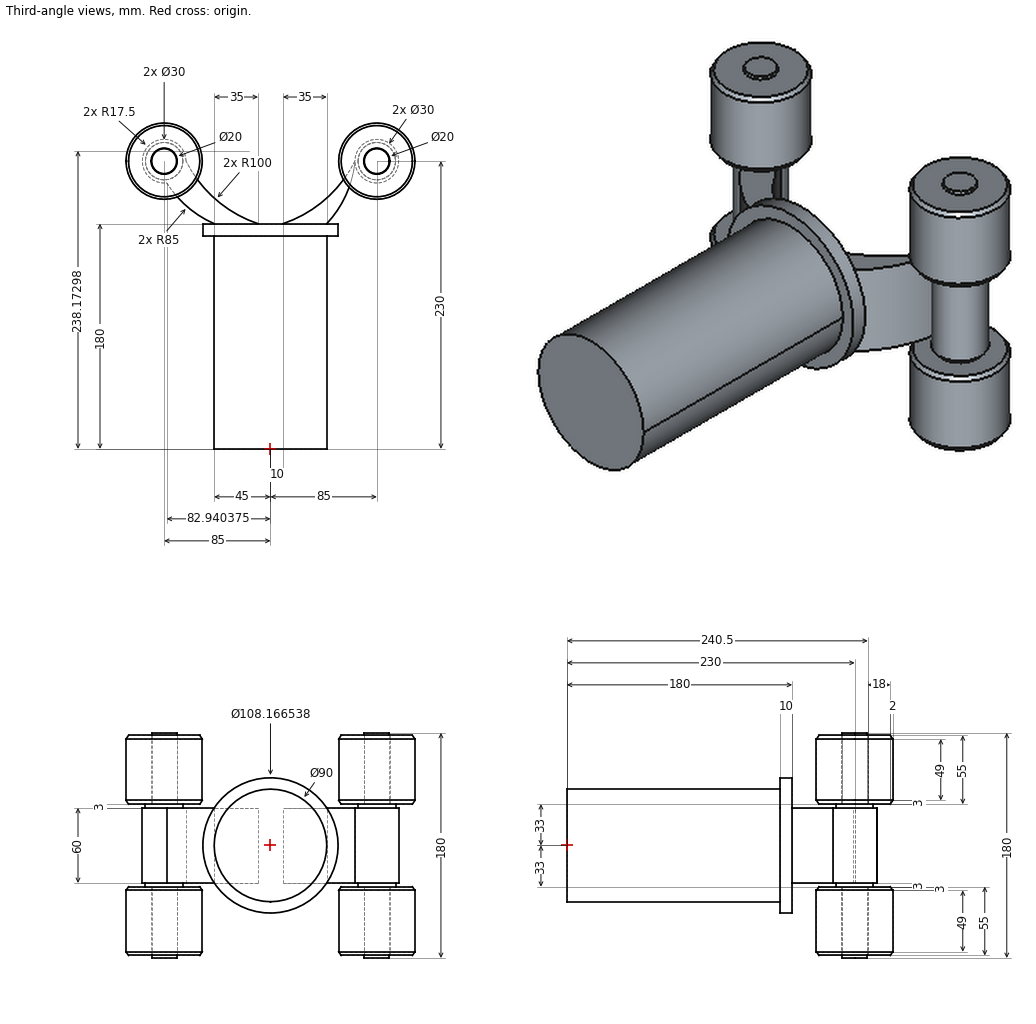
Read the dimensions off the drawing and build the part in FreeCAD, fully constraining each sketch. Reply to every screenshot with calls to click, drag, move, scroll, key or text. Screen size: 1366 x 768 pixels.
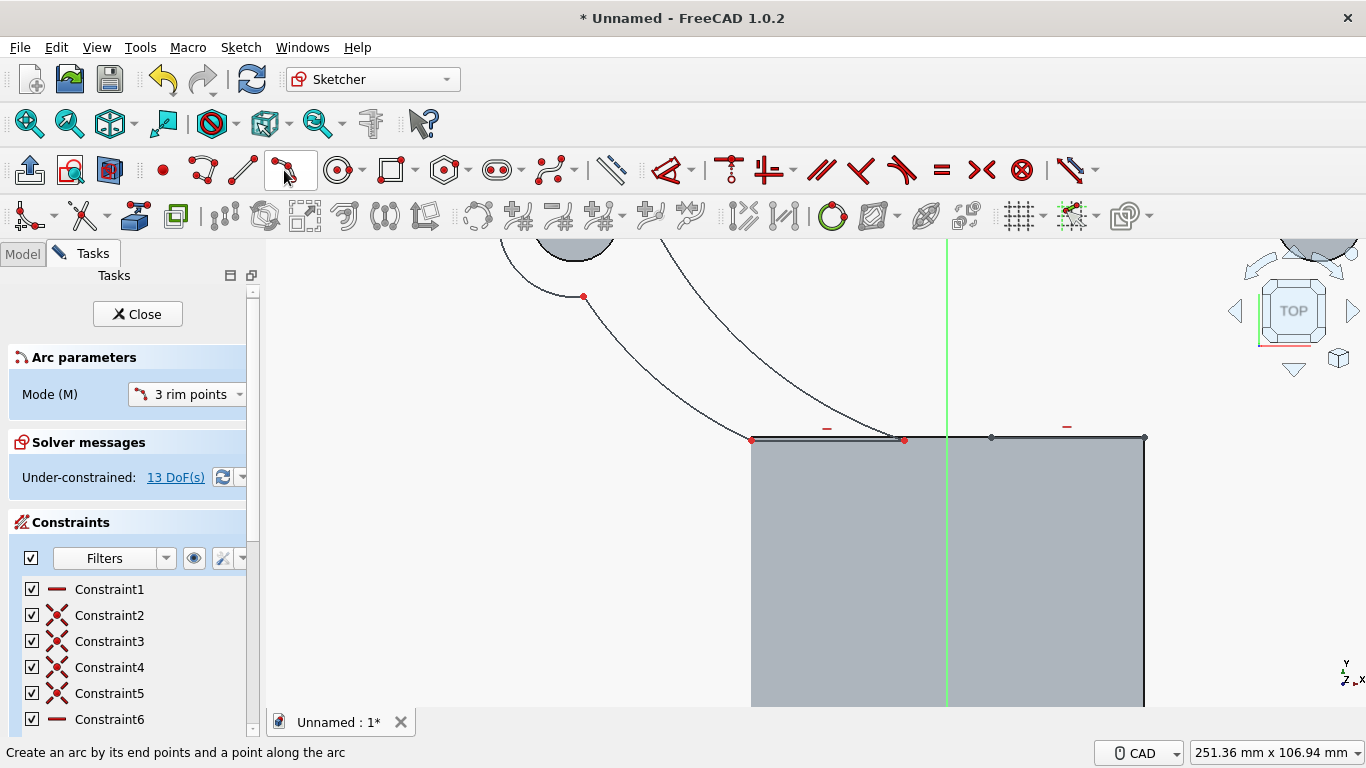
click(1144, 438)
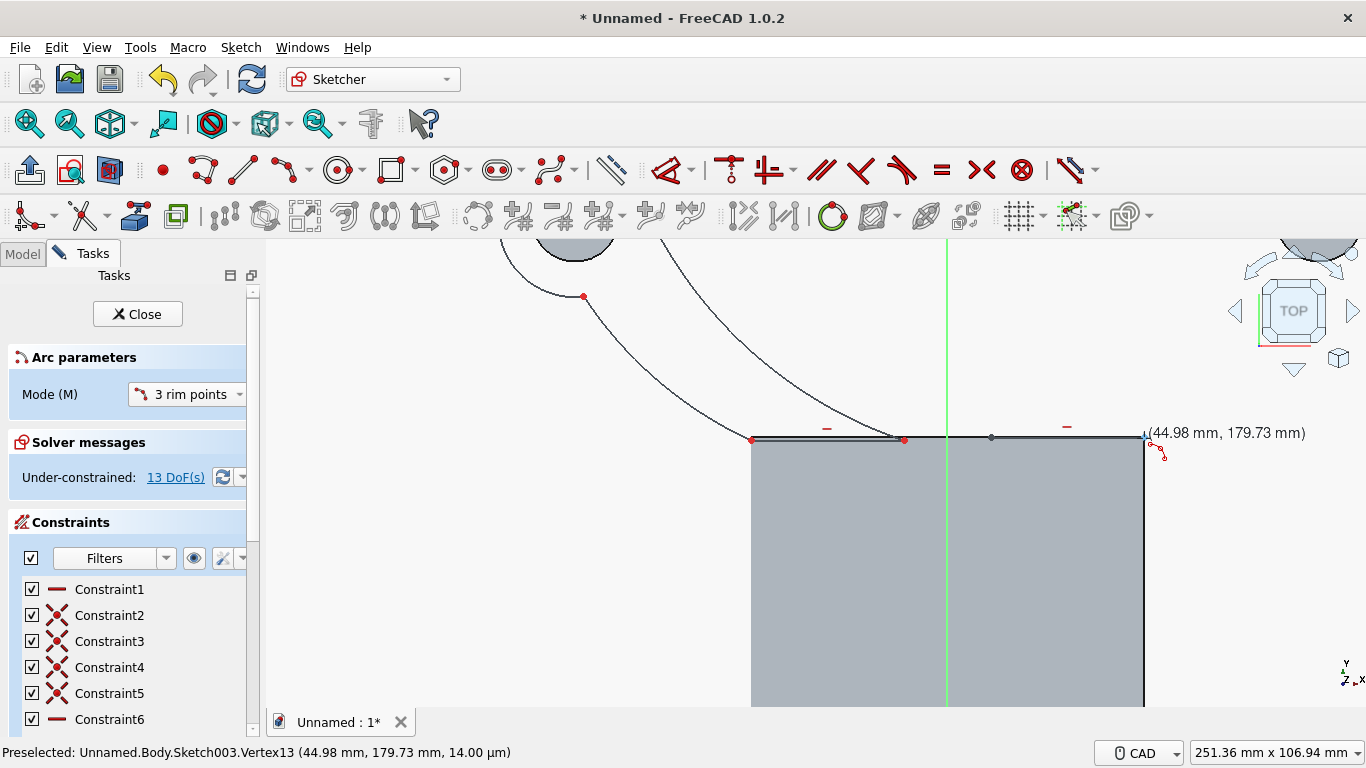
scroll(657, 377, down, 6)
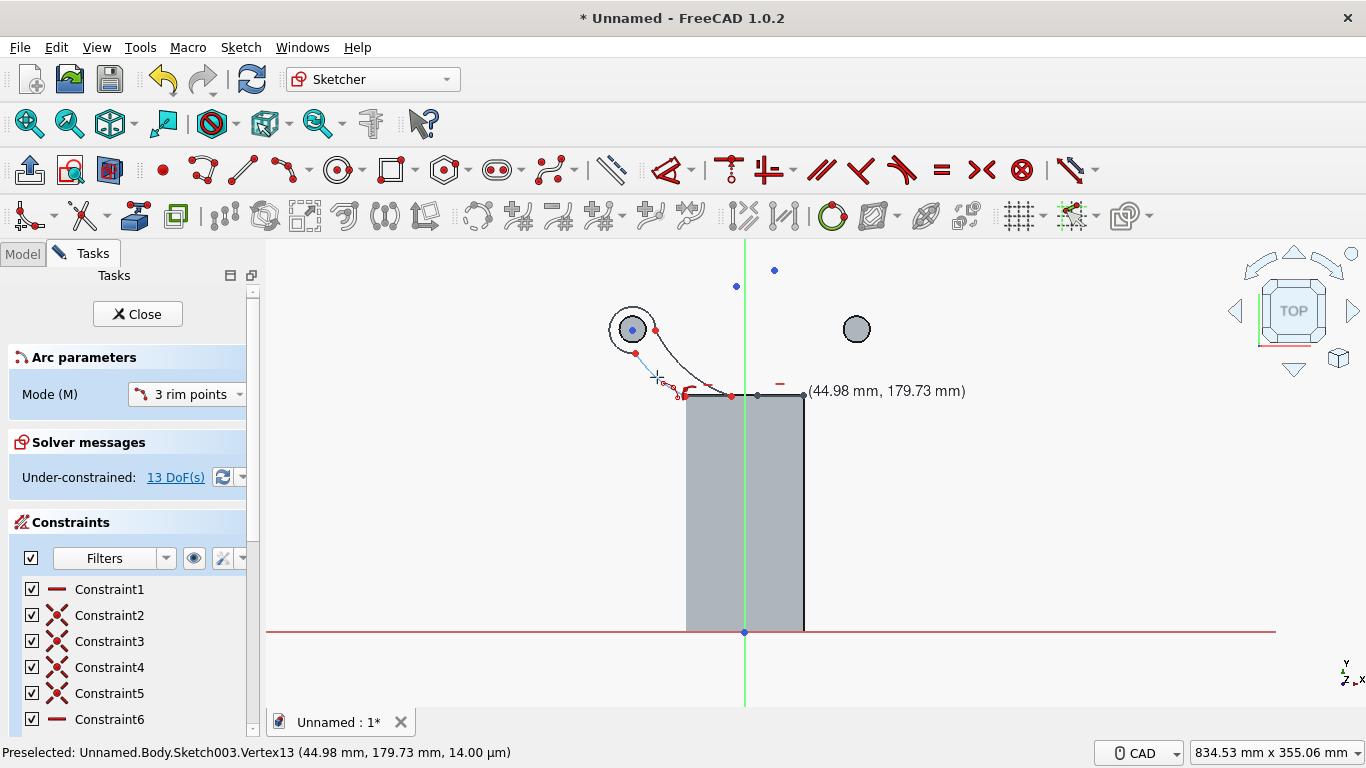
click(834, 331)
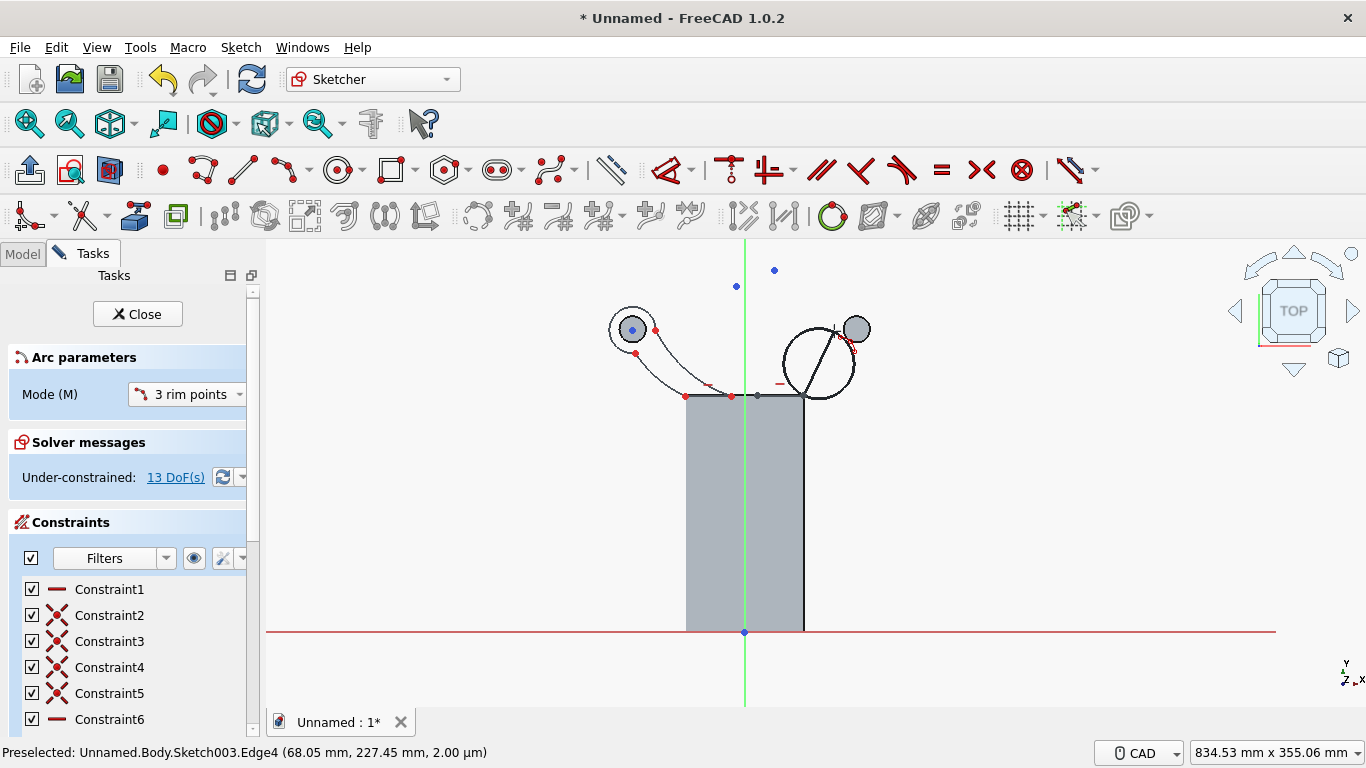
scroll(824, 365, up, 6)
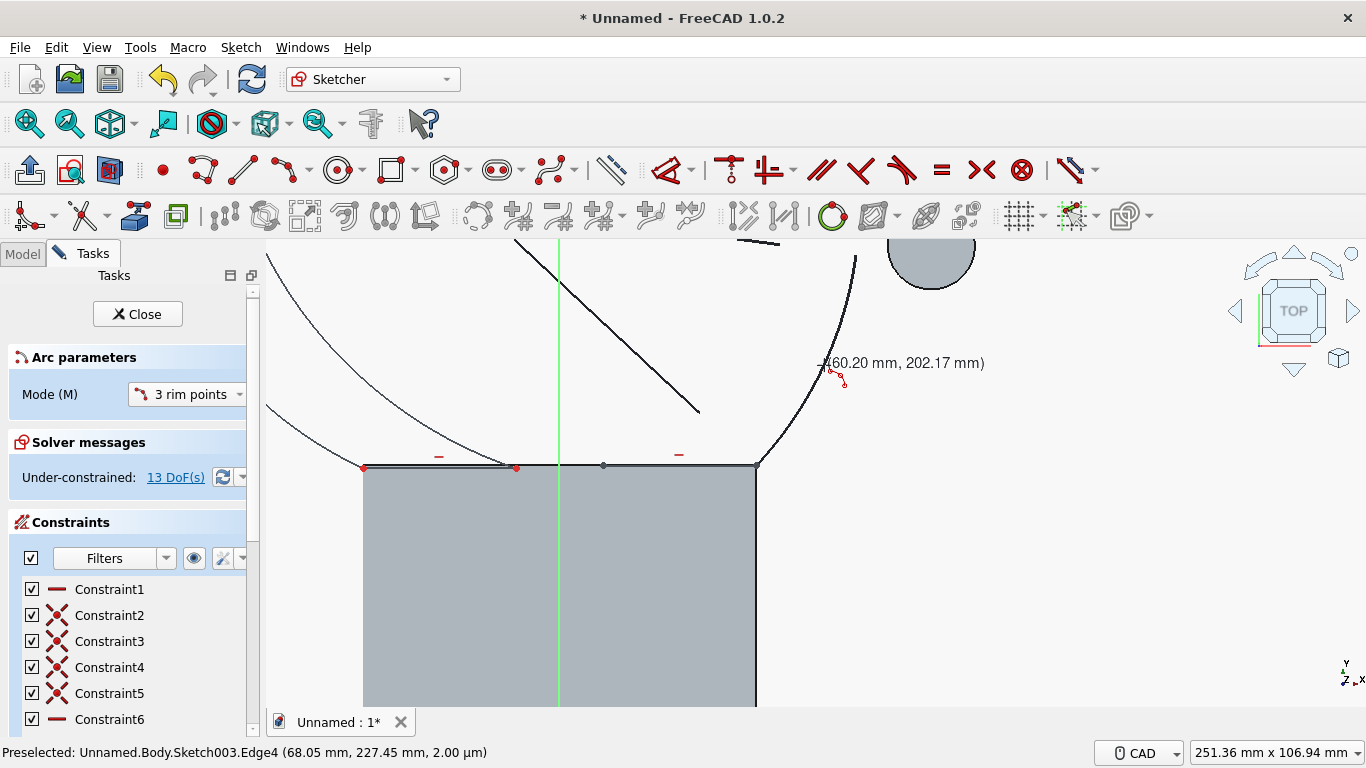
click(823, 366)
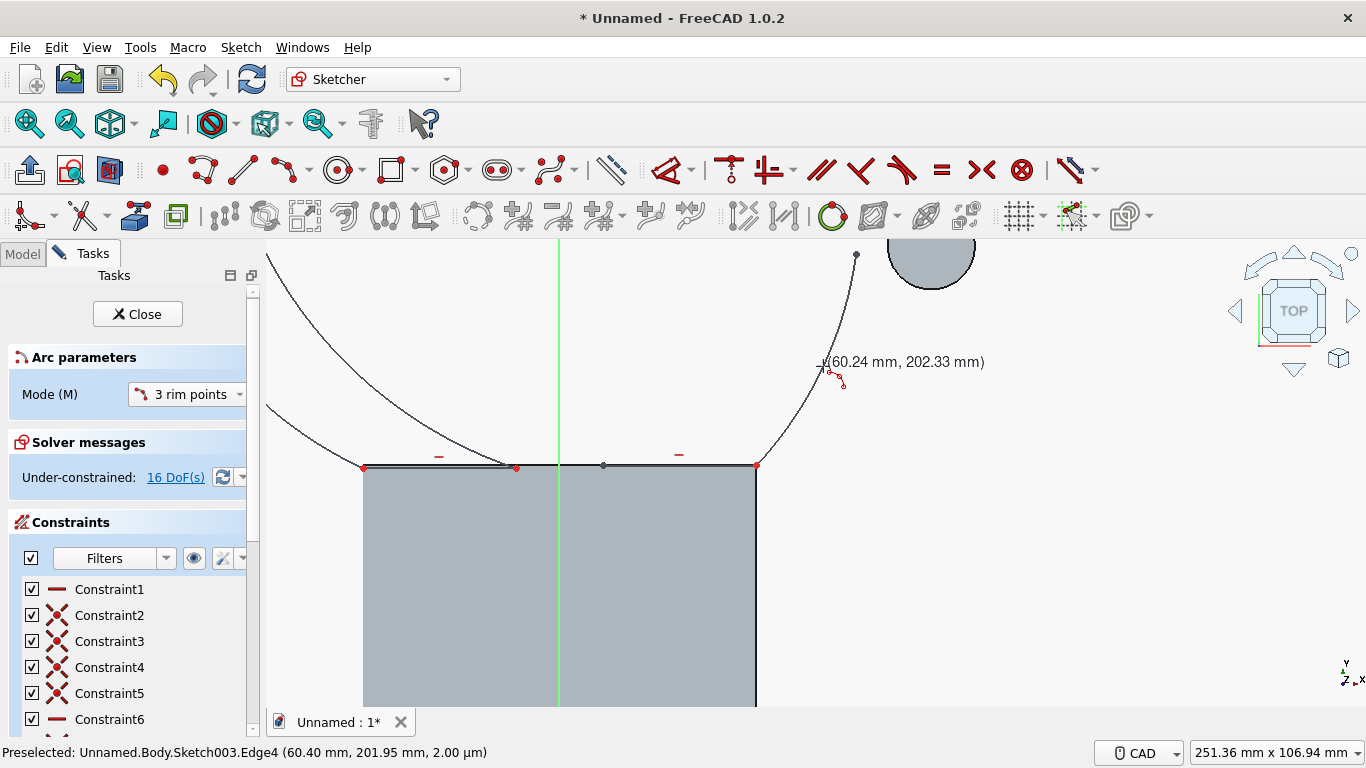
scroll(824, 365, down, 6)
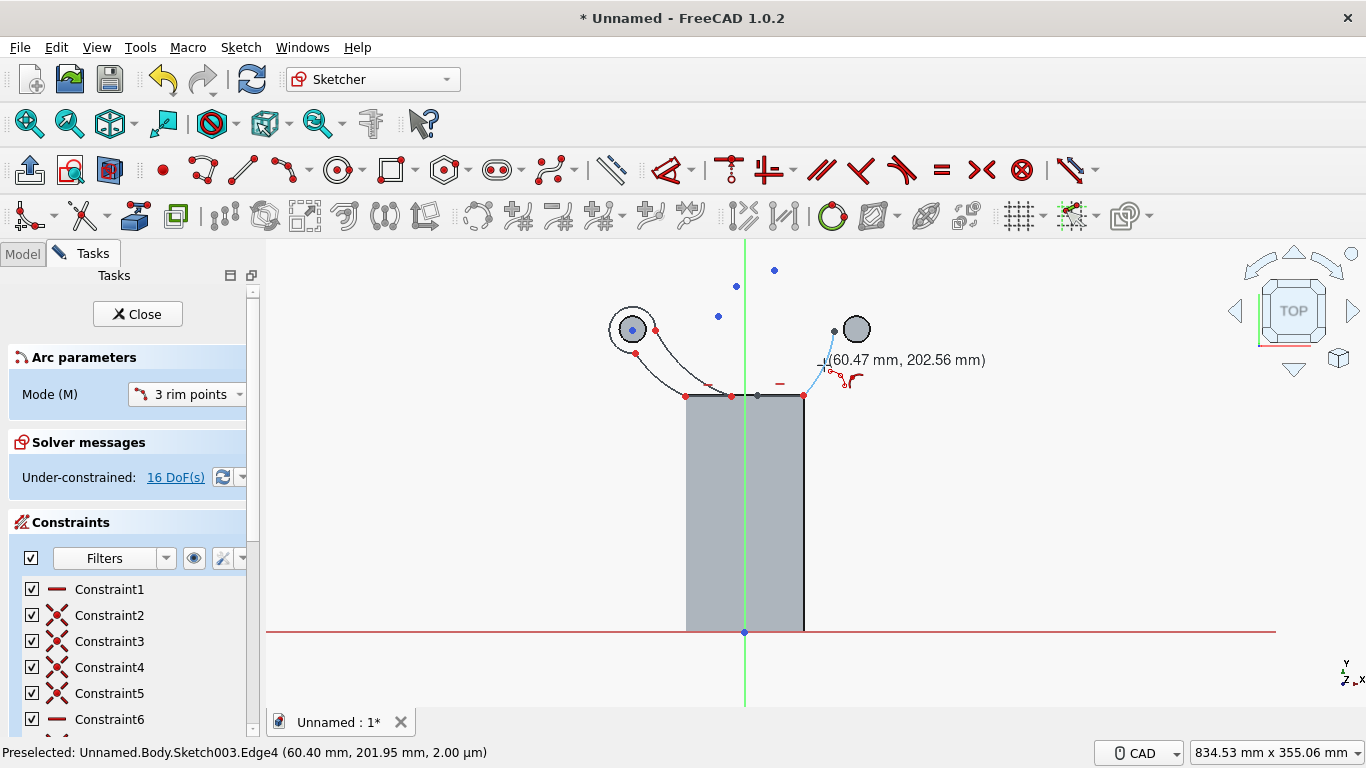
click(834, 332)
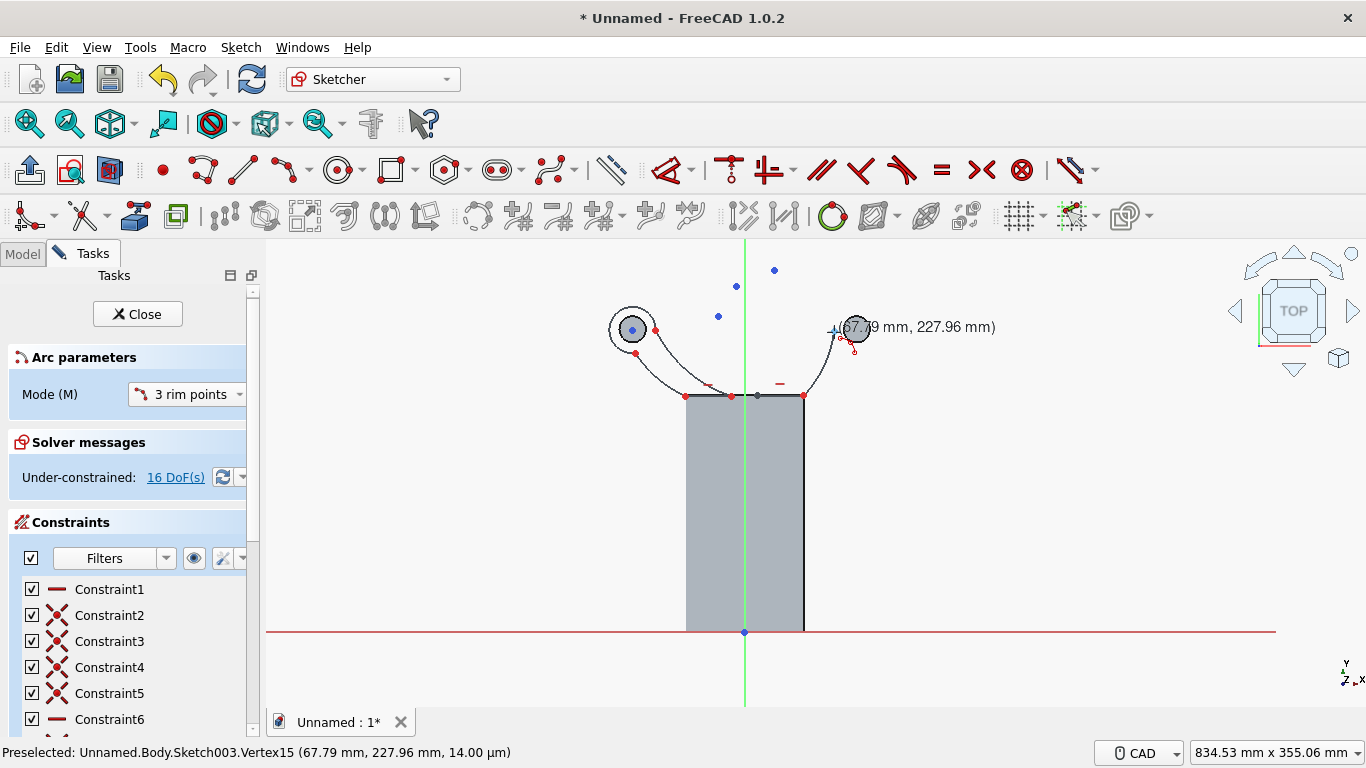
scroll(834, 329, up, 13)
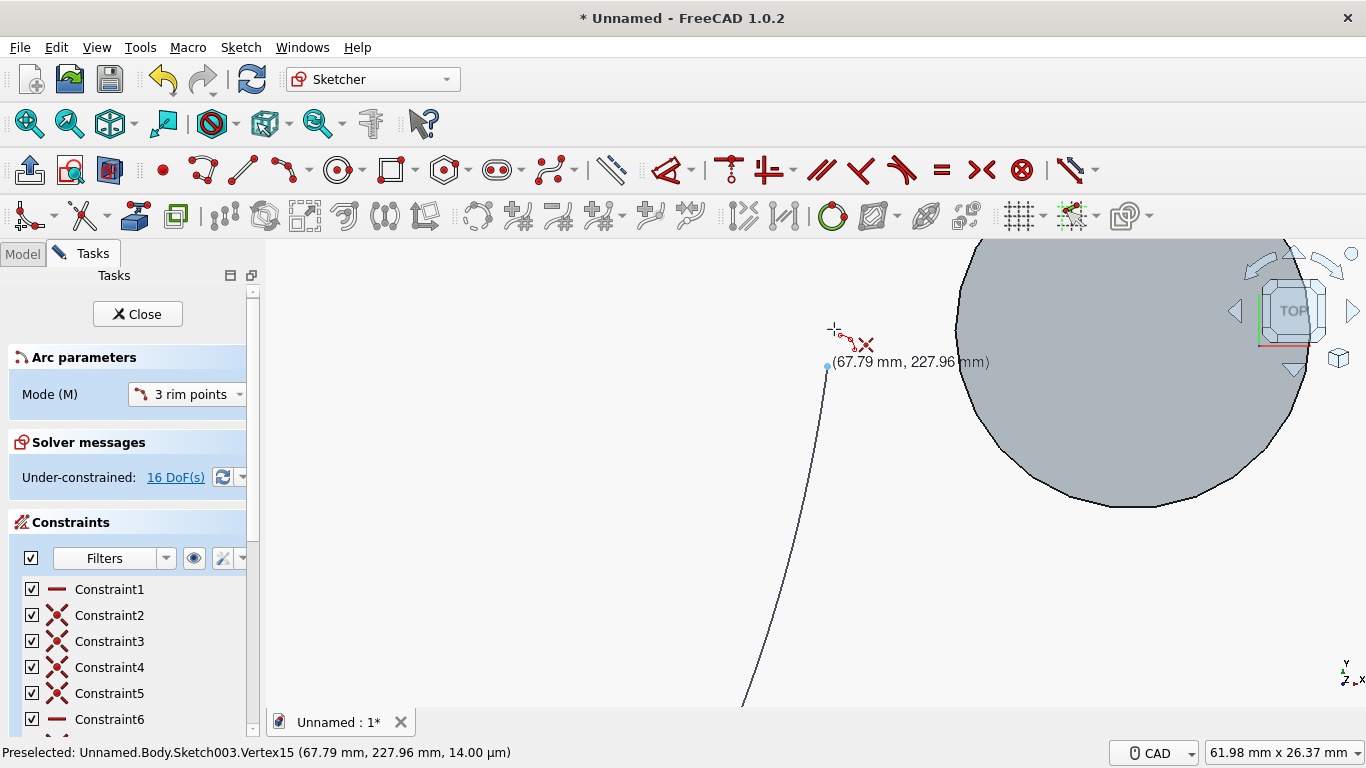
click(822, 331)